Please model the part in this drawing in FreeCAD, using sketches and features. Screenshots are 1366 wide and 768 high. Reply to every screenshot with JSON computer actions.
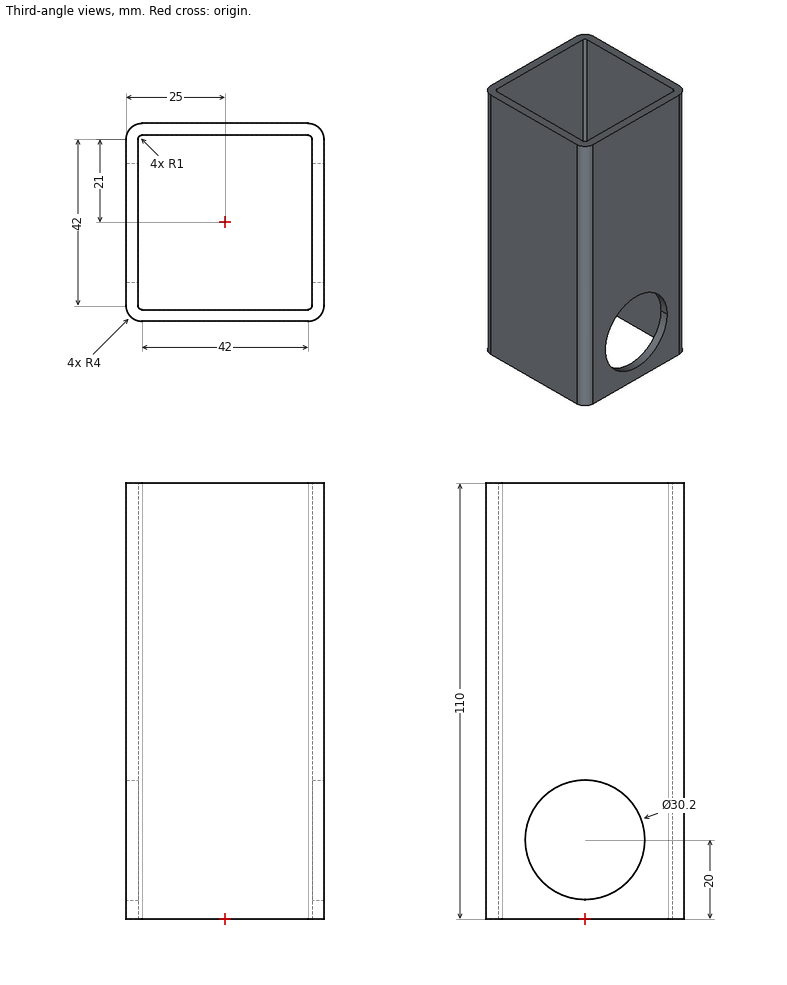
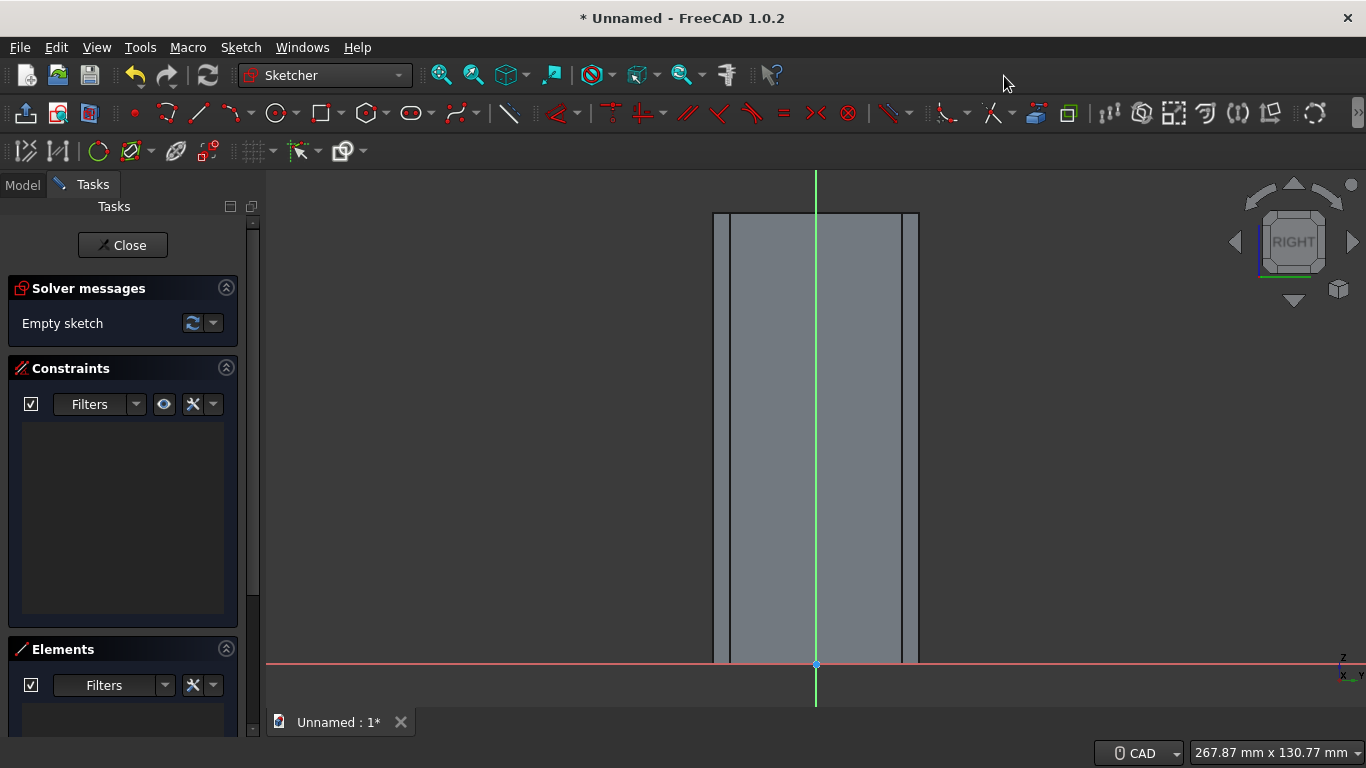
{"action": "scroll", "coordinate": [872, 679], "scroll_direction": "up", "scroll_amount": 4}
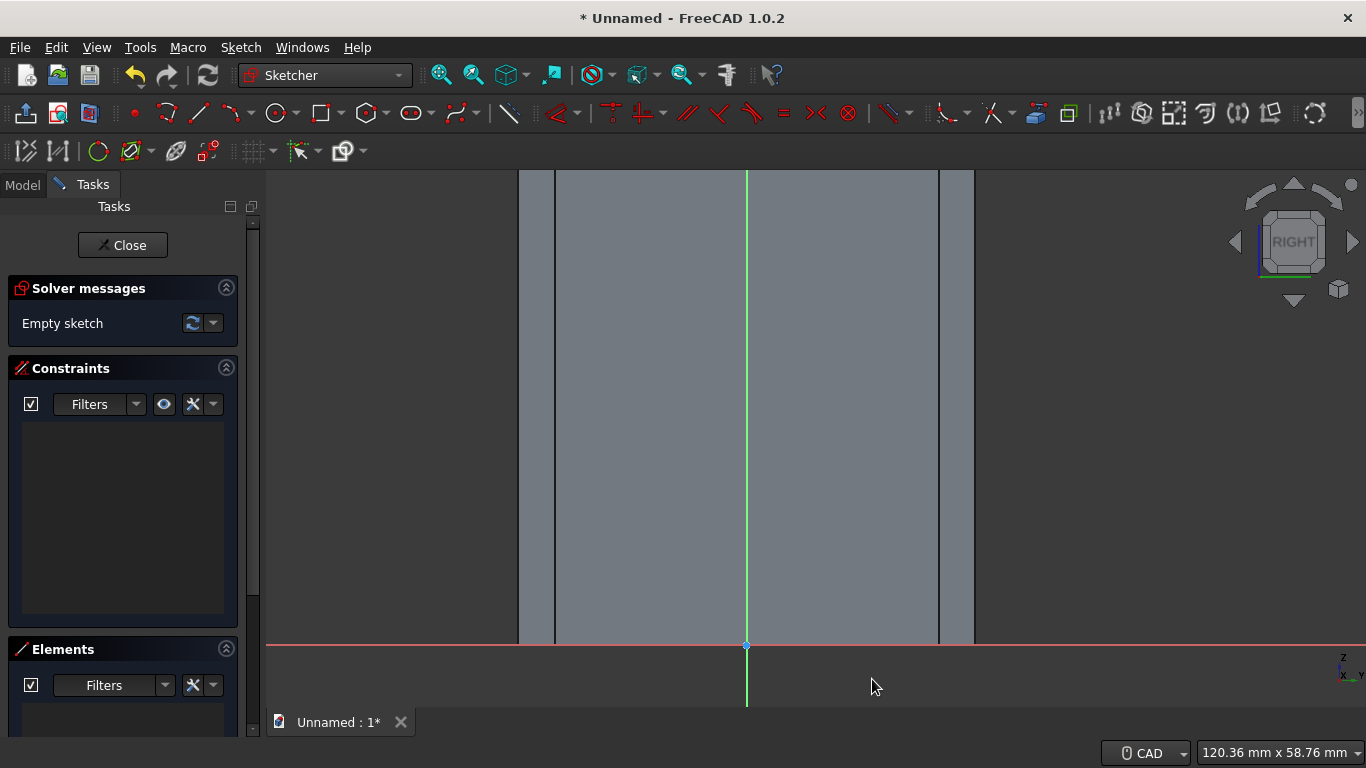
{"action": "left_click", "coordinate": [276, 114]}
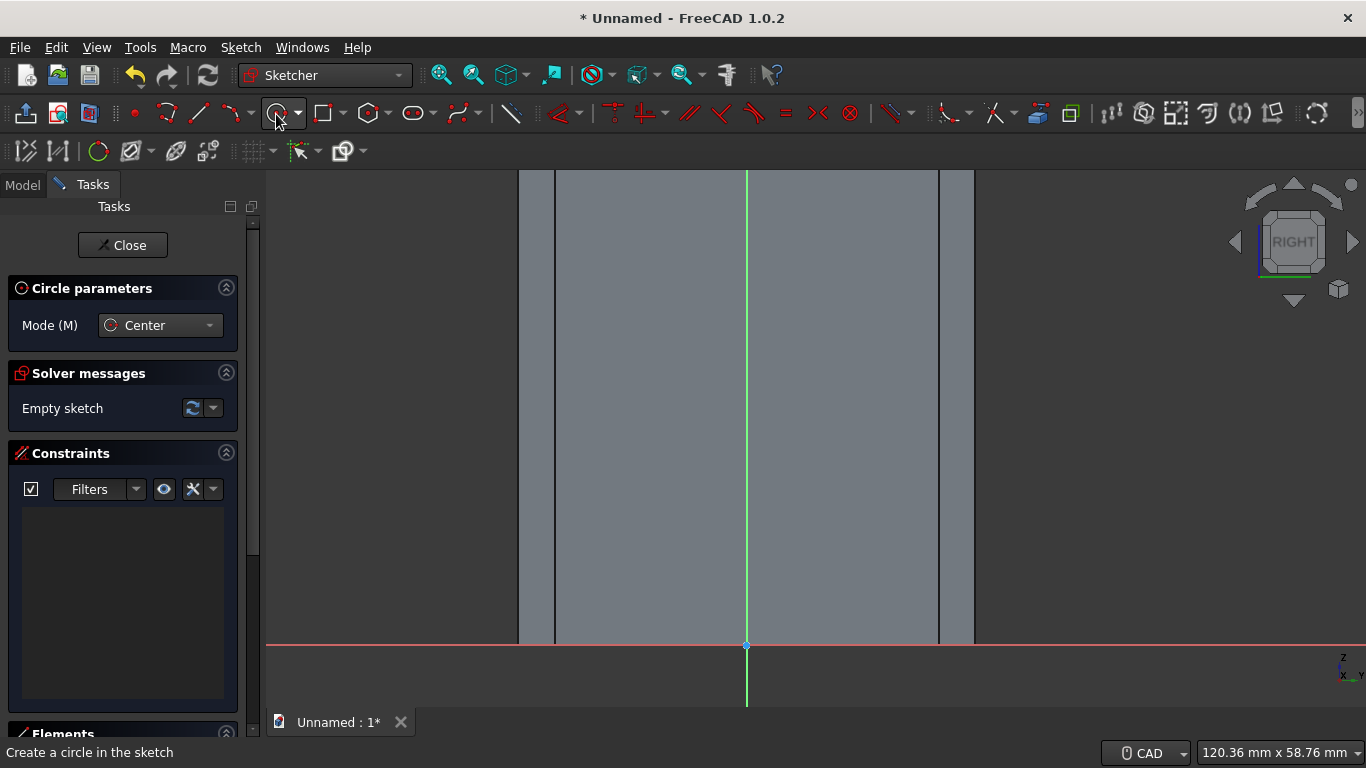
{"action": "left_click", "coordinate": [747, 462]}
{"action": "left_click", "coordinate": [844, 365]}
{"action": "key", "text": "Escape"}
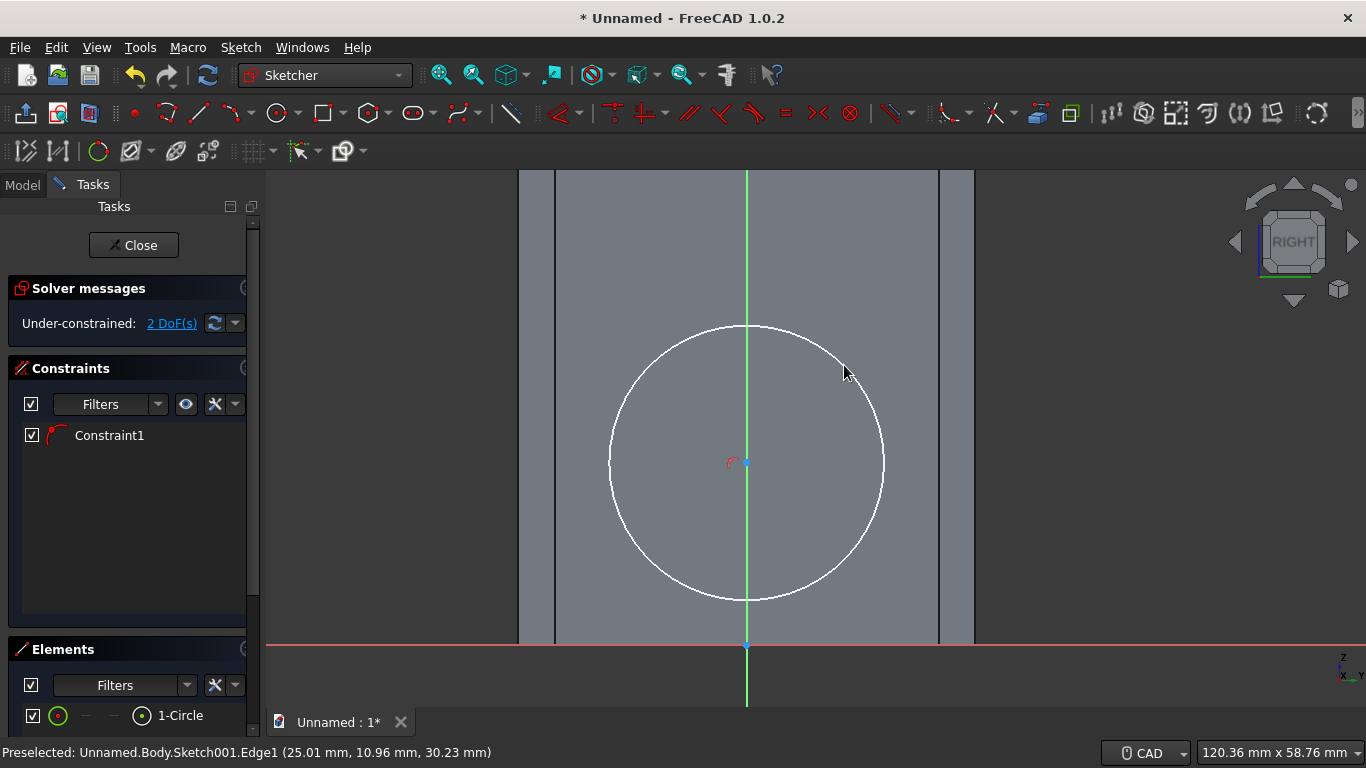
{"action": "left_click", "coordinate": [558, 114]}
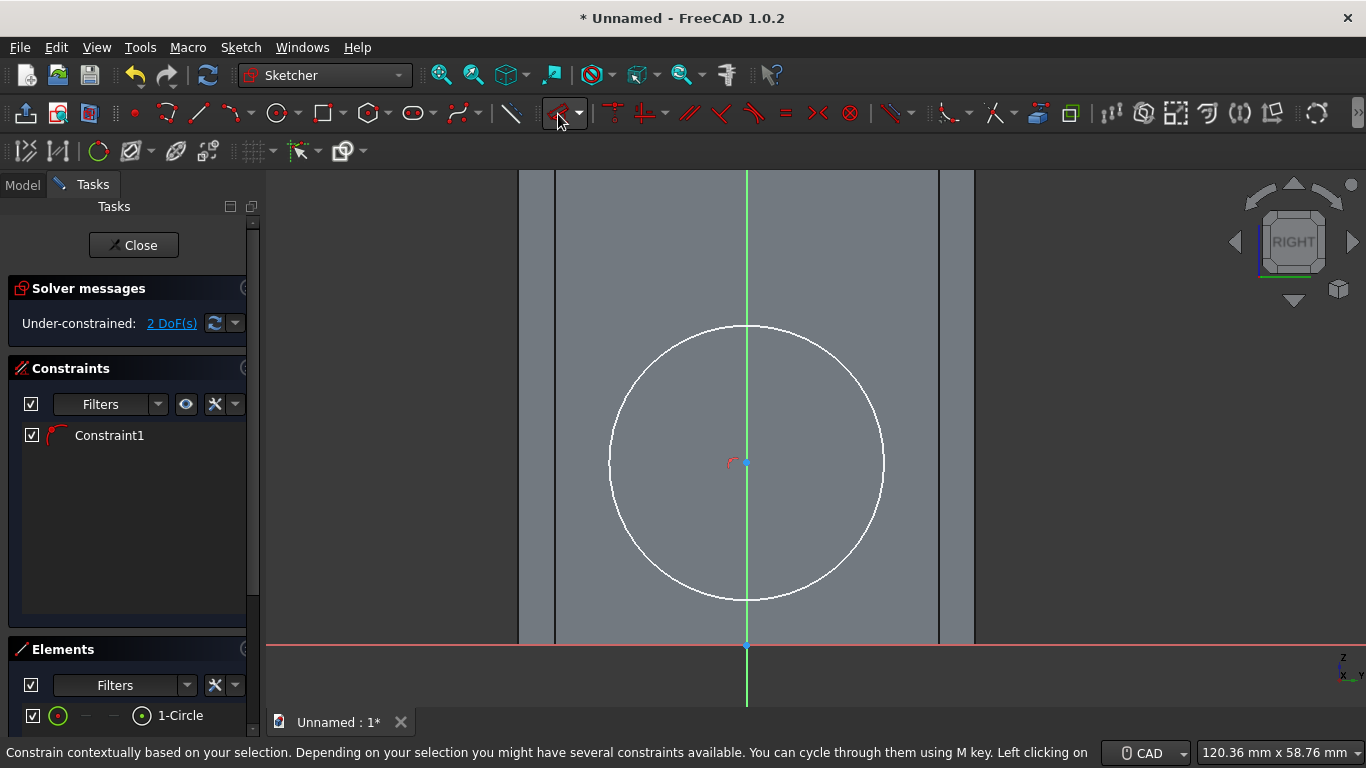
{"action": "left_click", "coordinate": [844, 366]}
{"action": "left_click", "coordinate": [867, 343]}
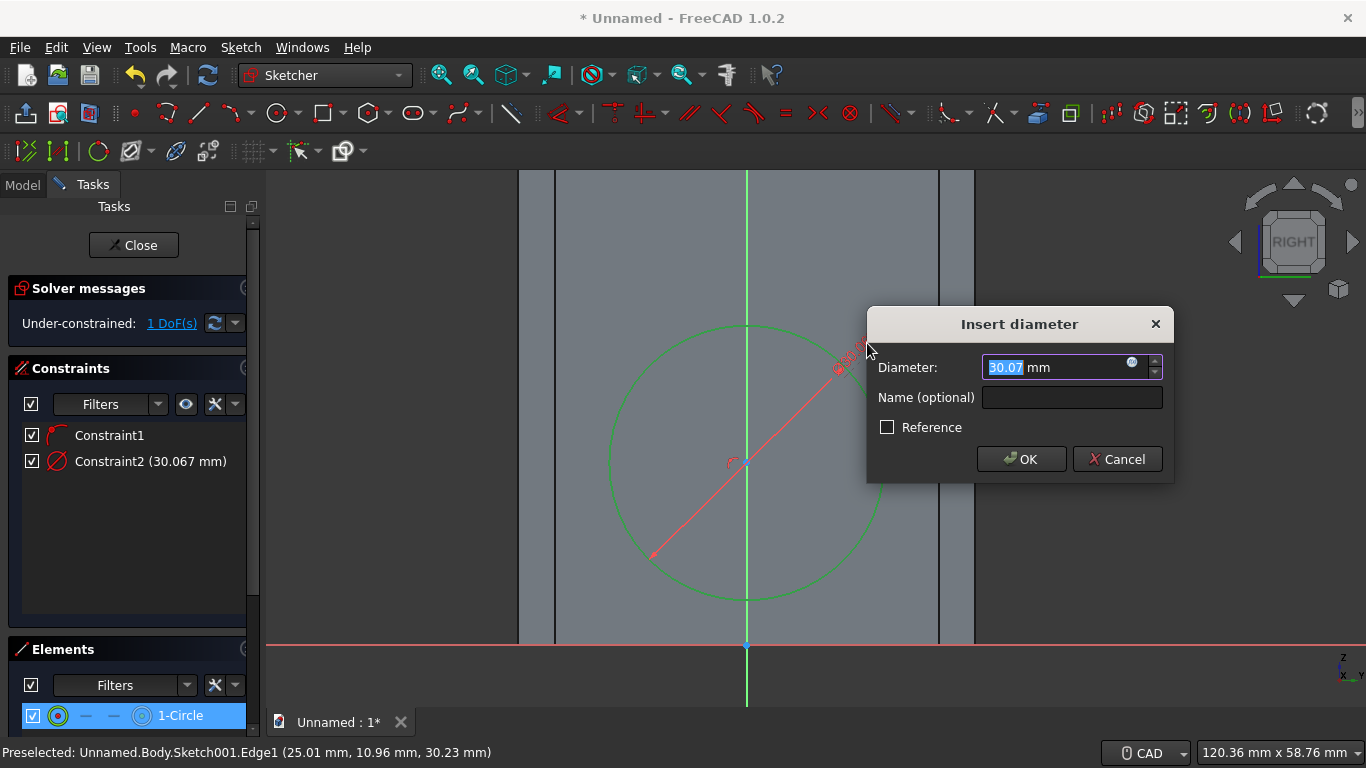
{"action": "type", "text": "30.2"}
{"action": "key", "text": "Return"}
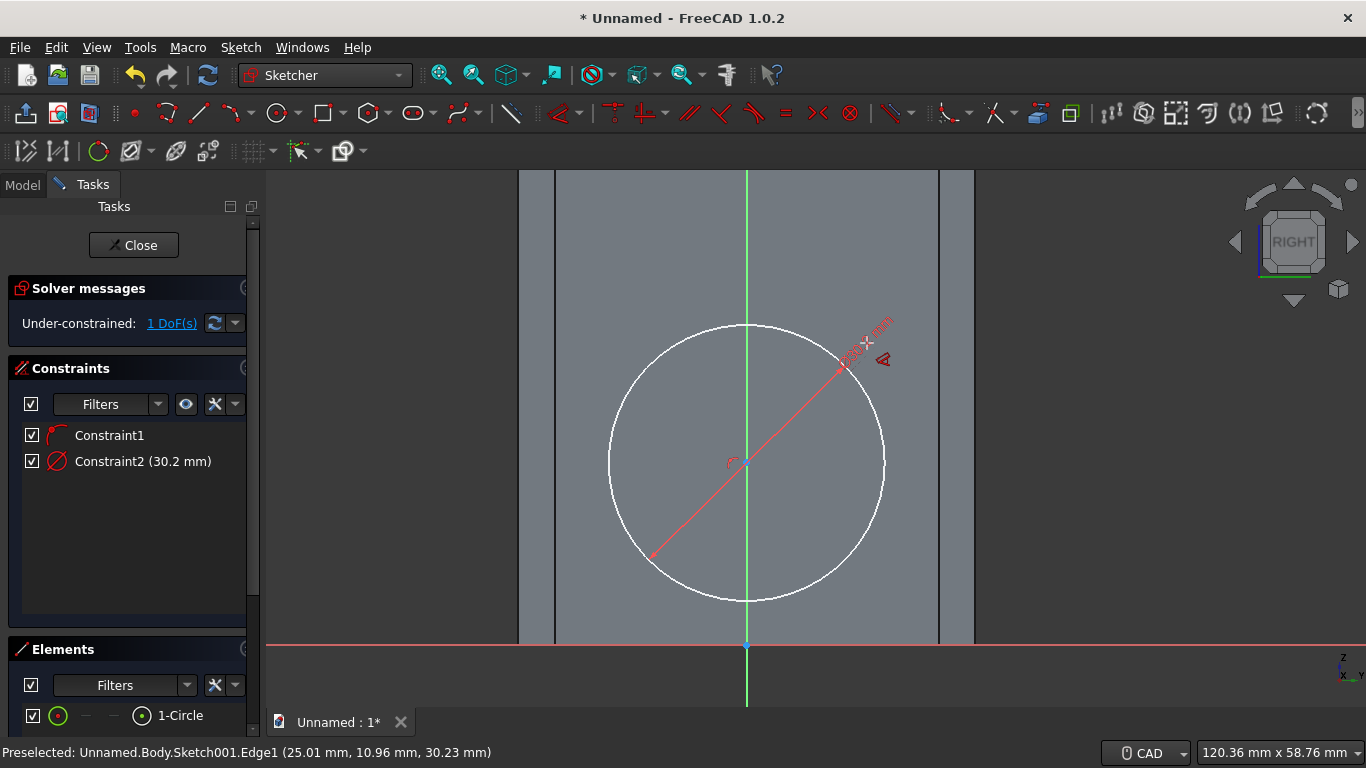
{"action": "left_click", "coordinate": [747, 463]}
{"action": "left_click", "coordinate": [781, 554]}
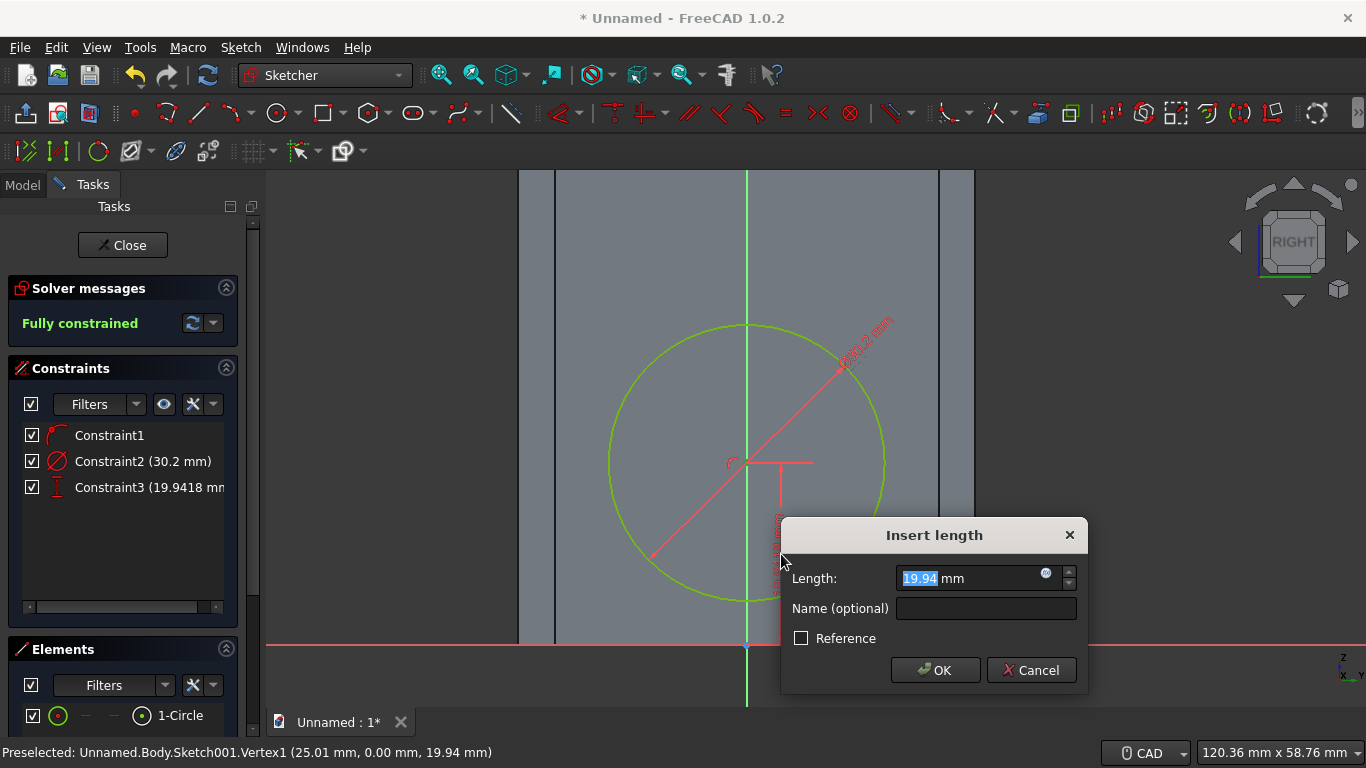
{"action": "type", "text": "20"}
{"action": "key", "text": "Return"}
{"action": "key", "text": "Escape"}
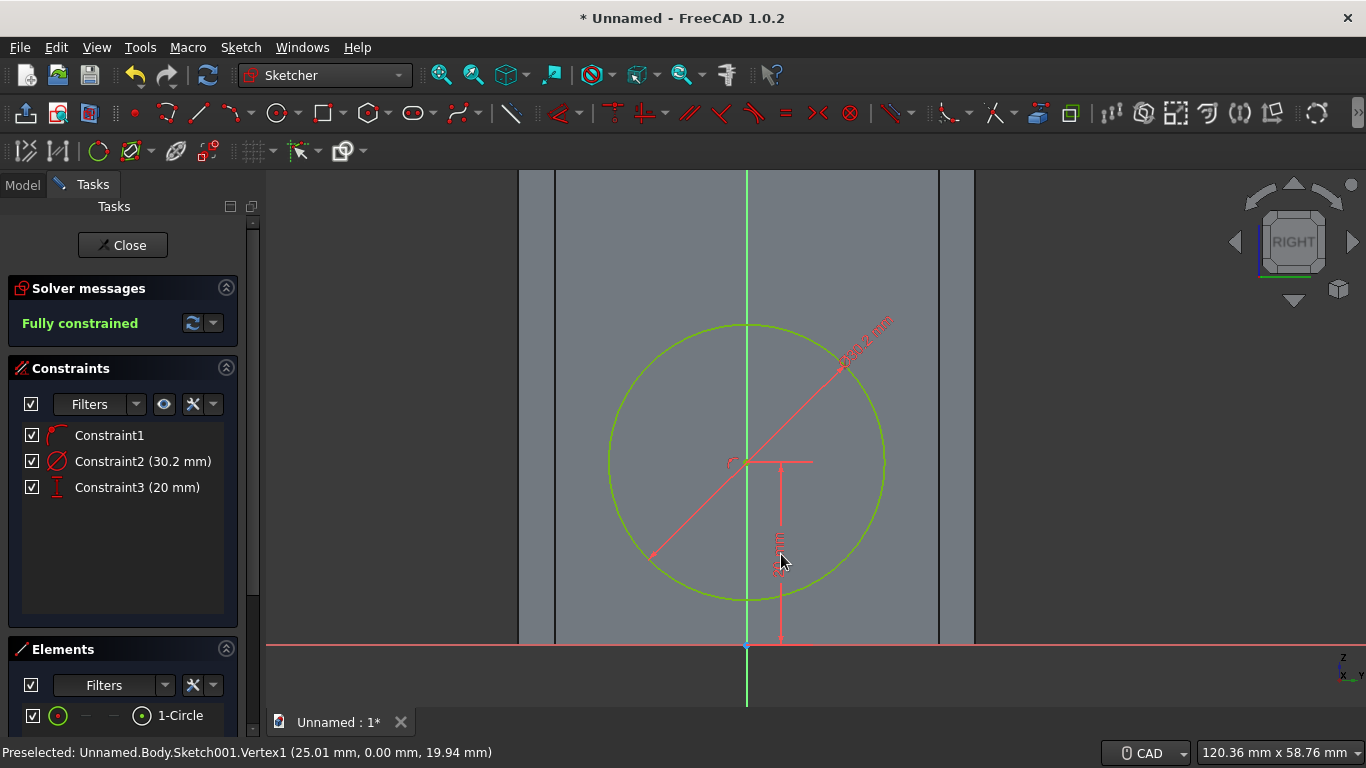
{"action": "left_click", "coordinate": [123, 245]}